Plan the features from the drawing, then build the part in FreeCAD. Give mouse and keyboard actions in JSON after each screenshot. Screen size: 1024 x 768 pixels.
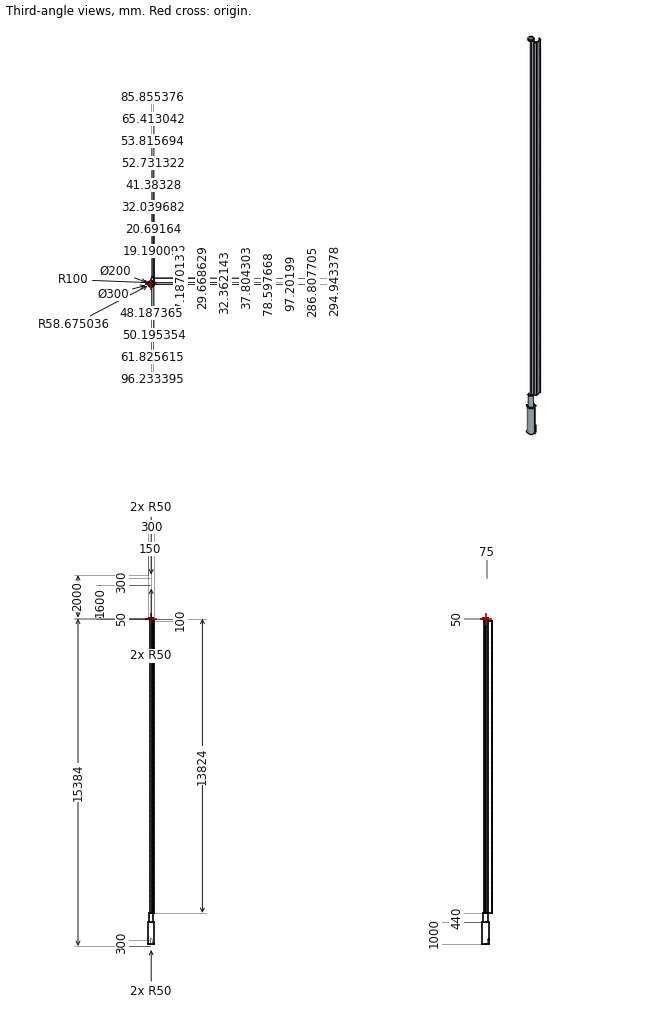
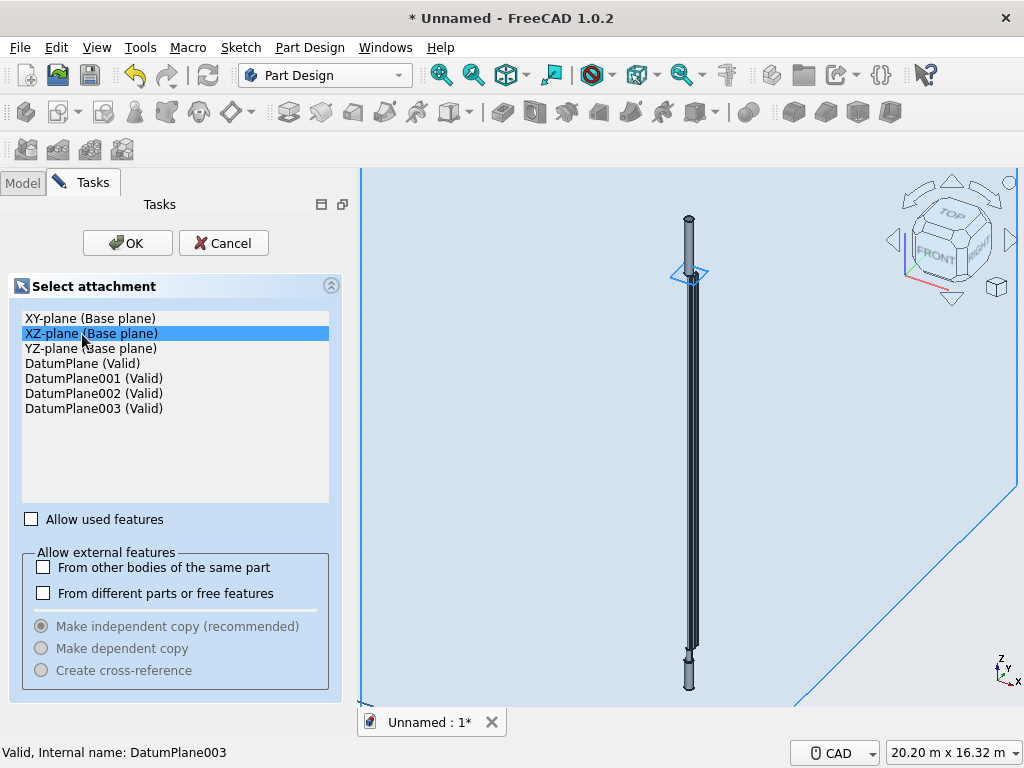
{"action": "left_click", "coordinate": [128, 243]}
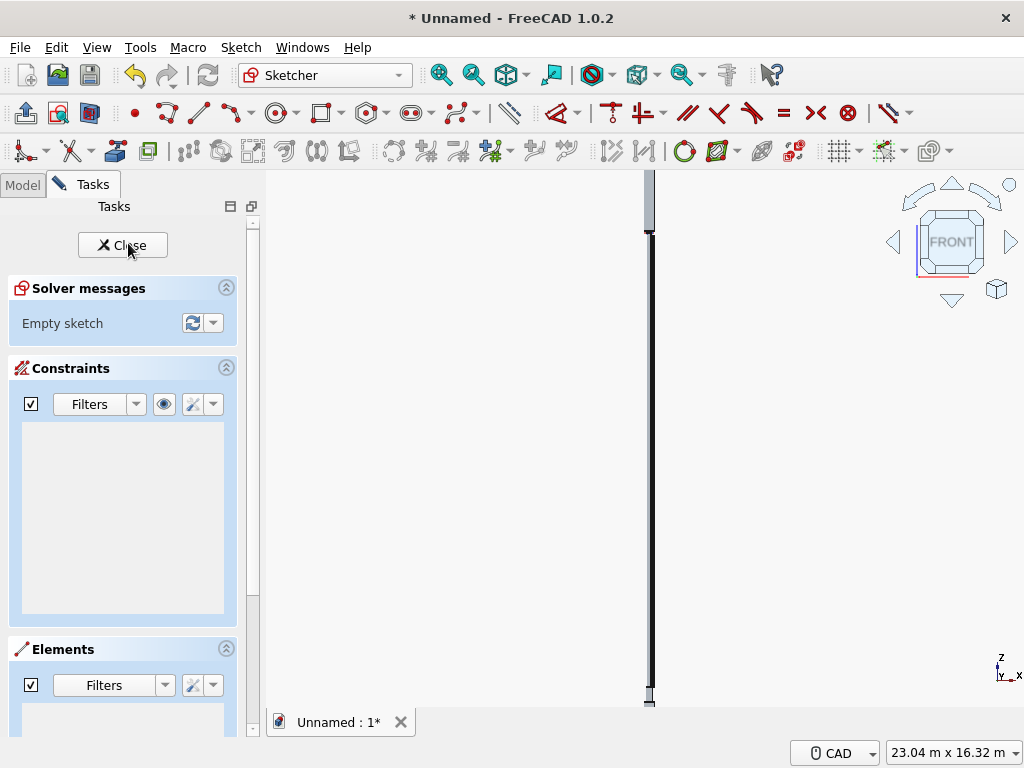
{"action": "left_click", "coordinate": [90, 114]}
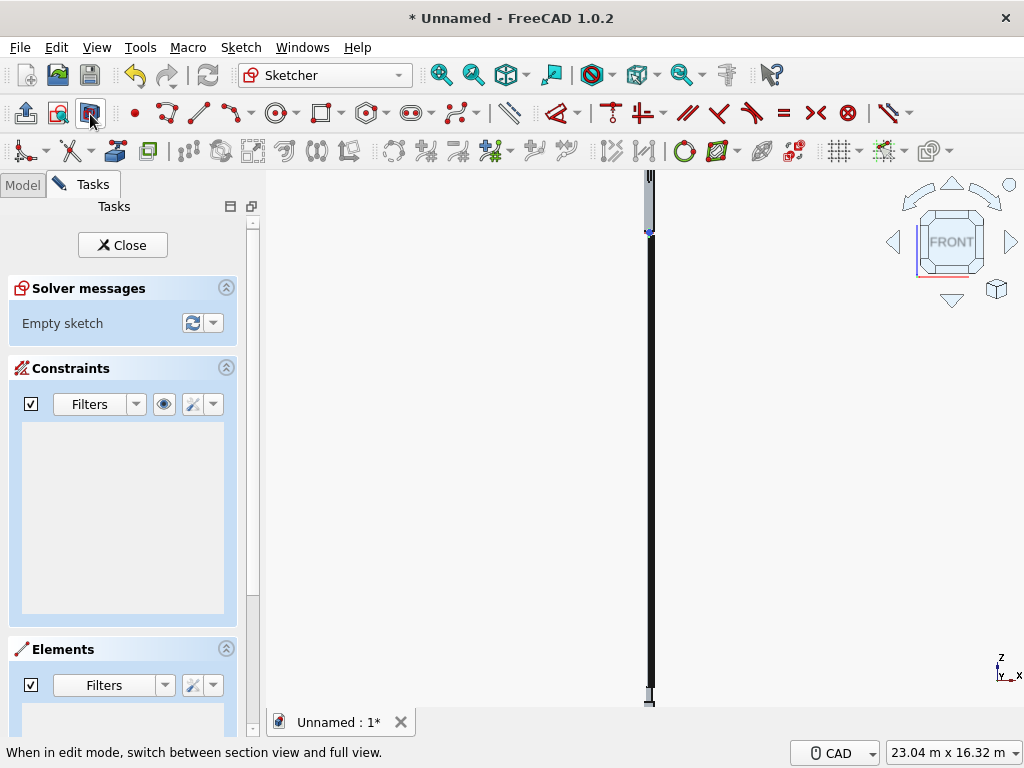
{"action": "scroll", "coordinate": [576, 438], "scroll_direction": "down", "scroll_amount": 5}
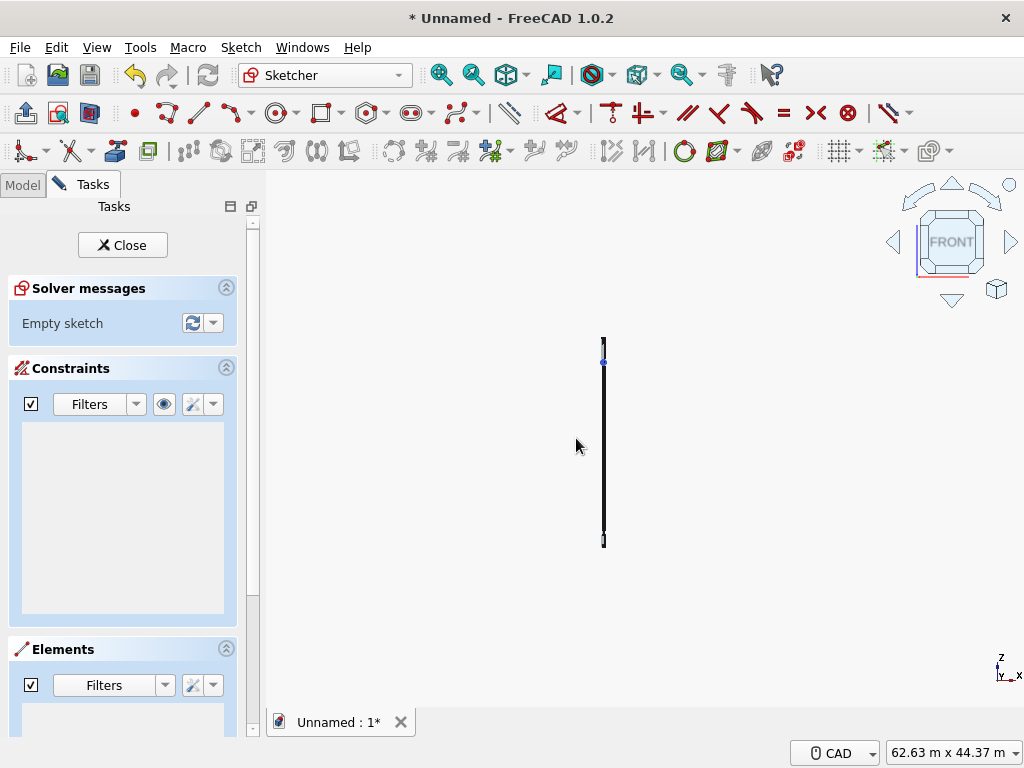
{"action": "scroll", "coordinate": [605, 343], "scroll_direction": "up", "scroll_amount": 13}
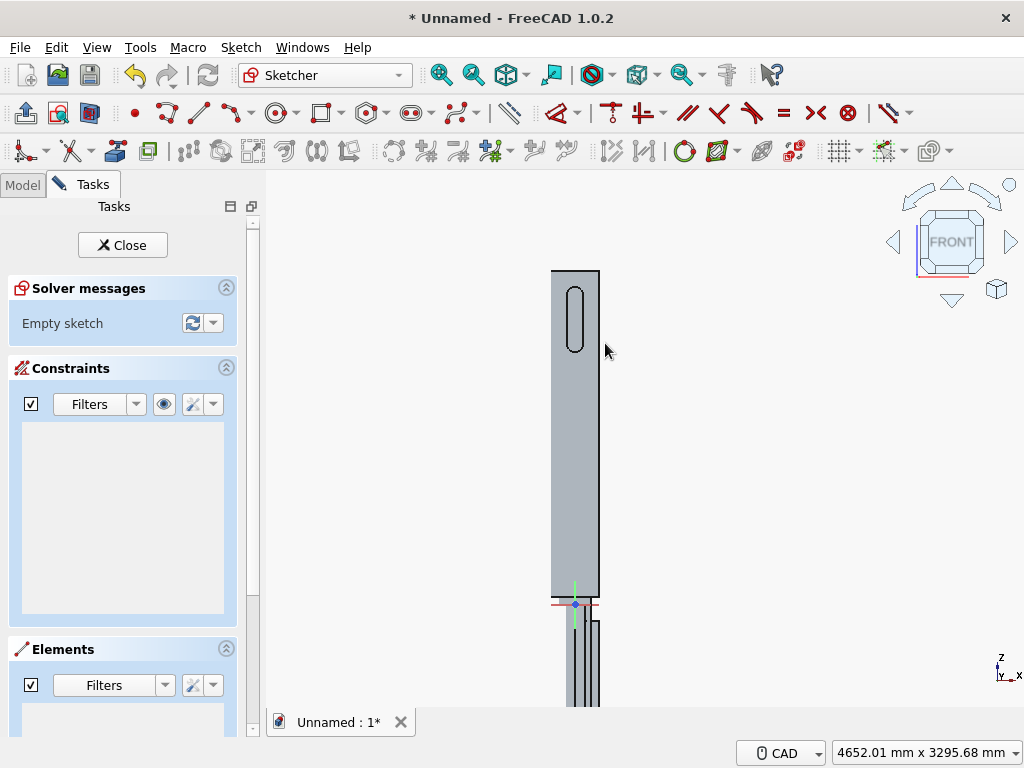
{"action": "left_click", "coordinate": [322, 114]}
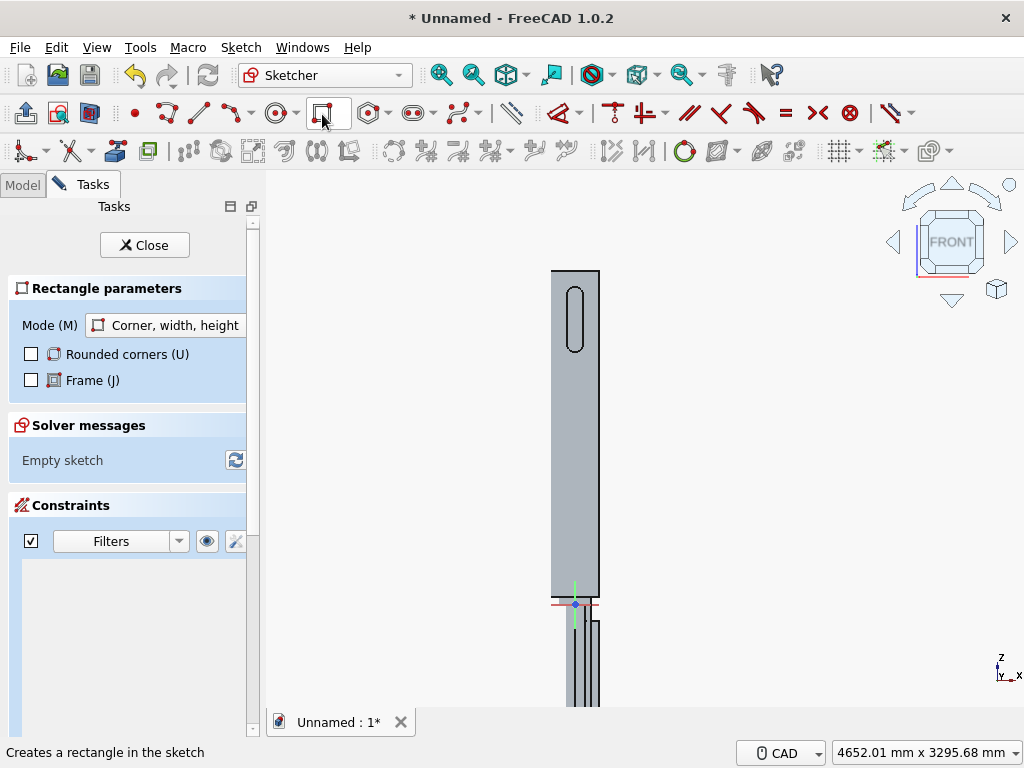
{"action": "left_click", "coordinate": [551, 271]}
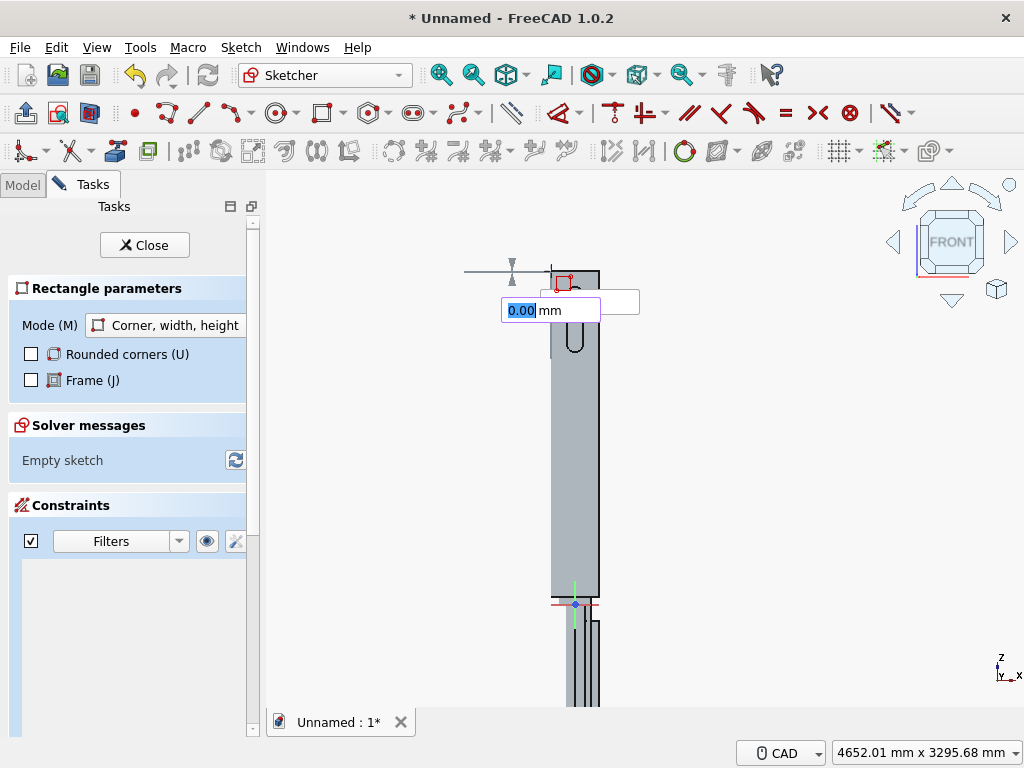
{"action": "scroll", "coordinate": [599, 597], "scroll_direction": "up", "scroll_amount": 4}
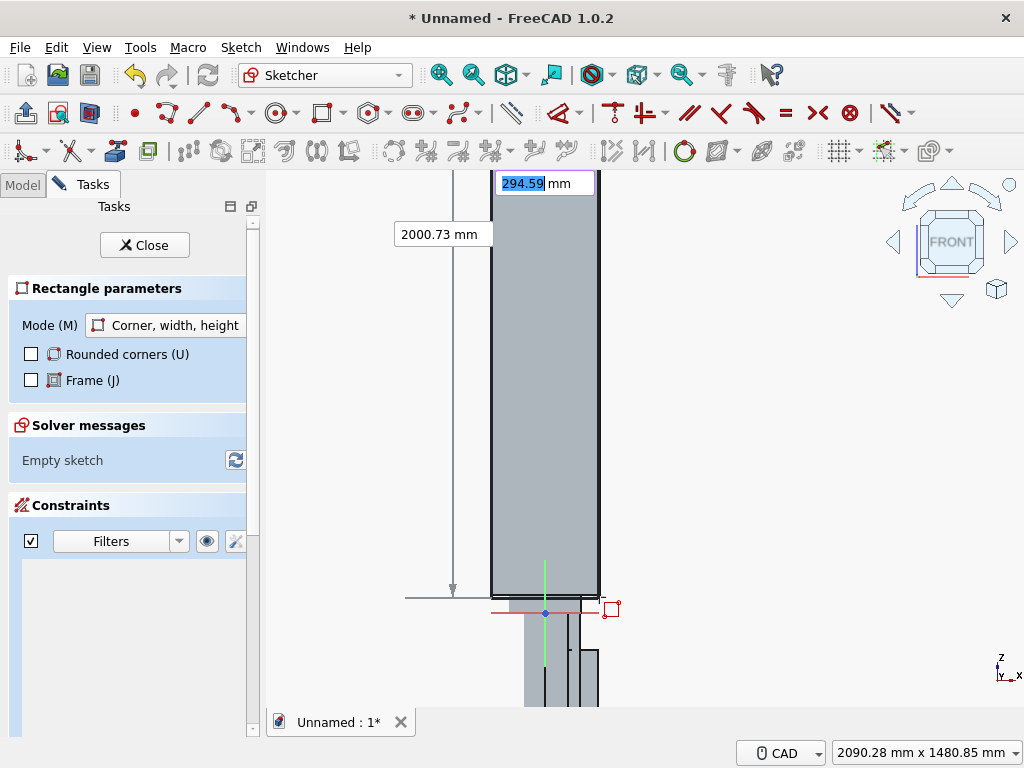
{"action": "left_click", "coordinate": [600, 595]}
{"action": "key", "text": "Escape"}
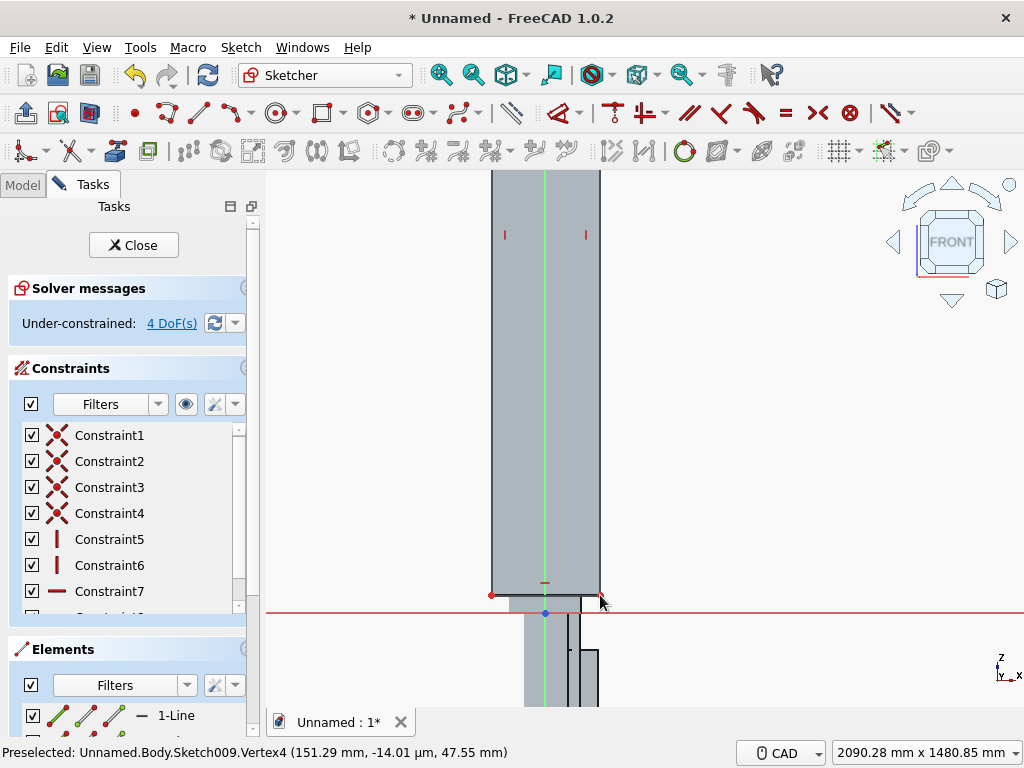
{"action": "left_click", "coordinate": [558, 114]}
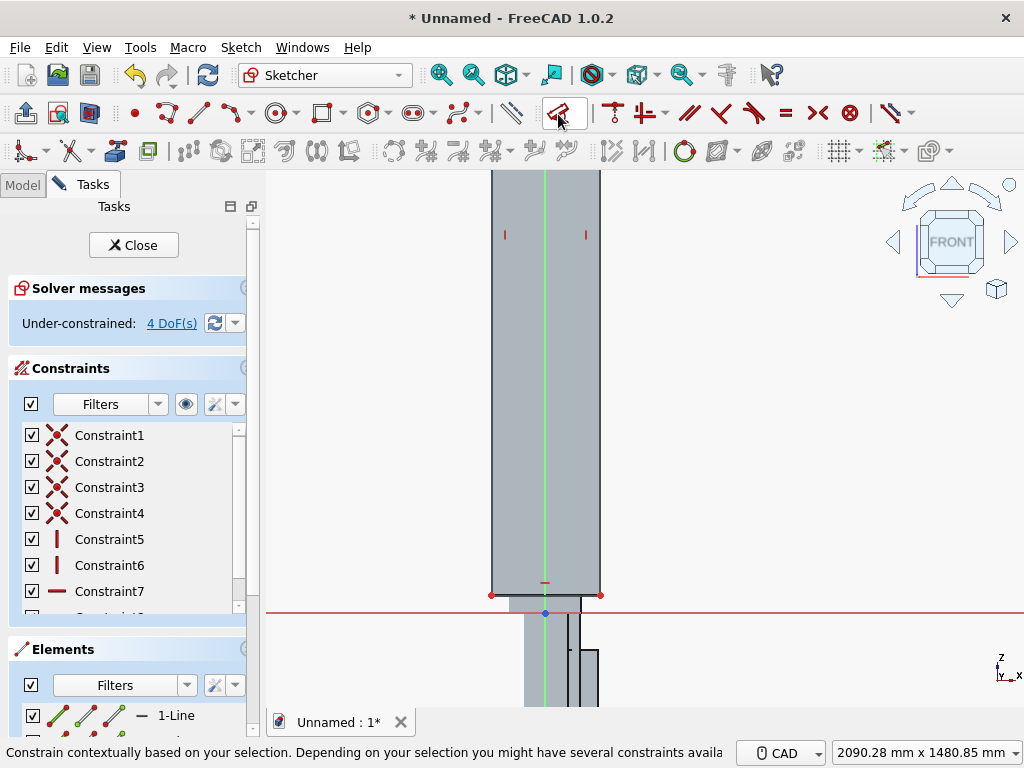
{"action": "left_click", "coordinate": [524, 596]}
{"action": "left_click", "coordinate": [521, 630]}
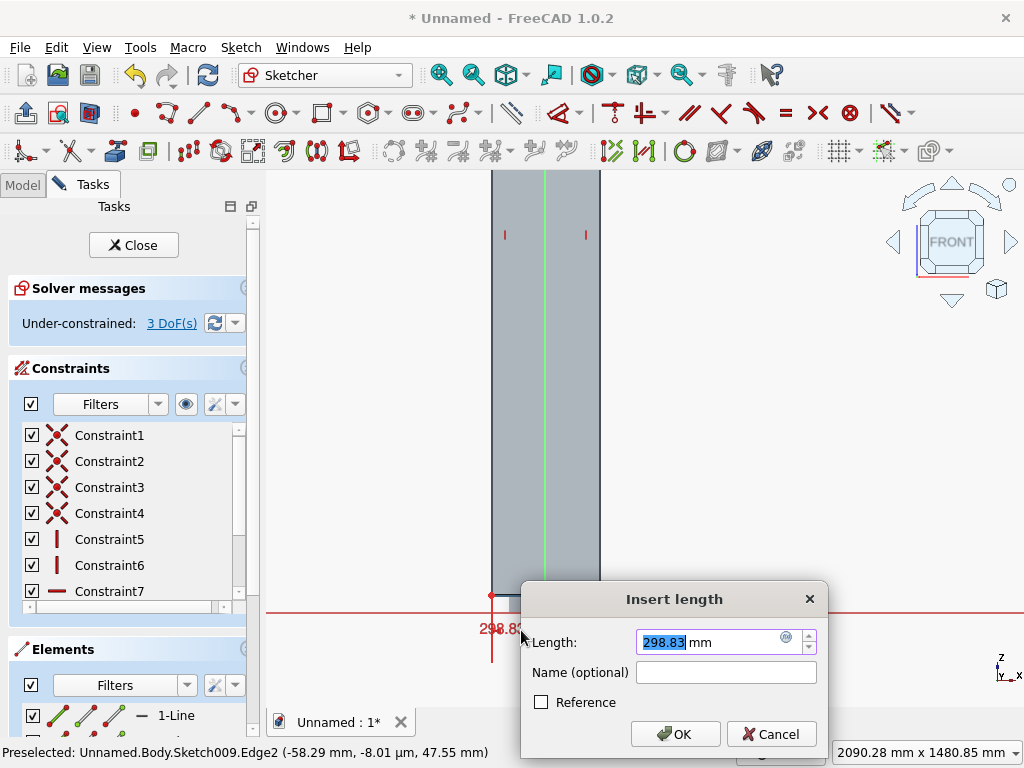
{"action": "type", "text": "300"}
{"action": "key", "text": "Return"}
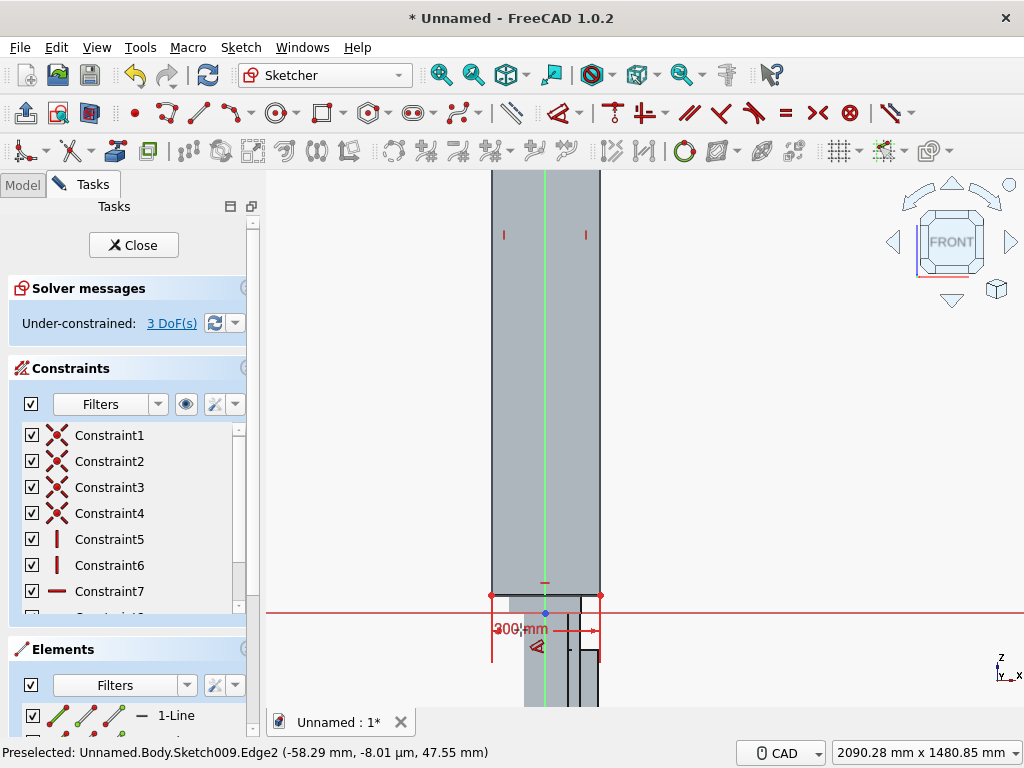
{"action": "scroll", "coordinate": [492, 596], "scroll_direction": "up", "scroll_amount": 4}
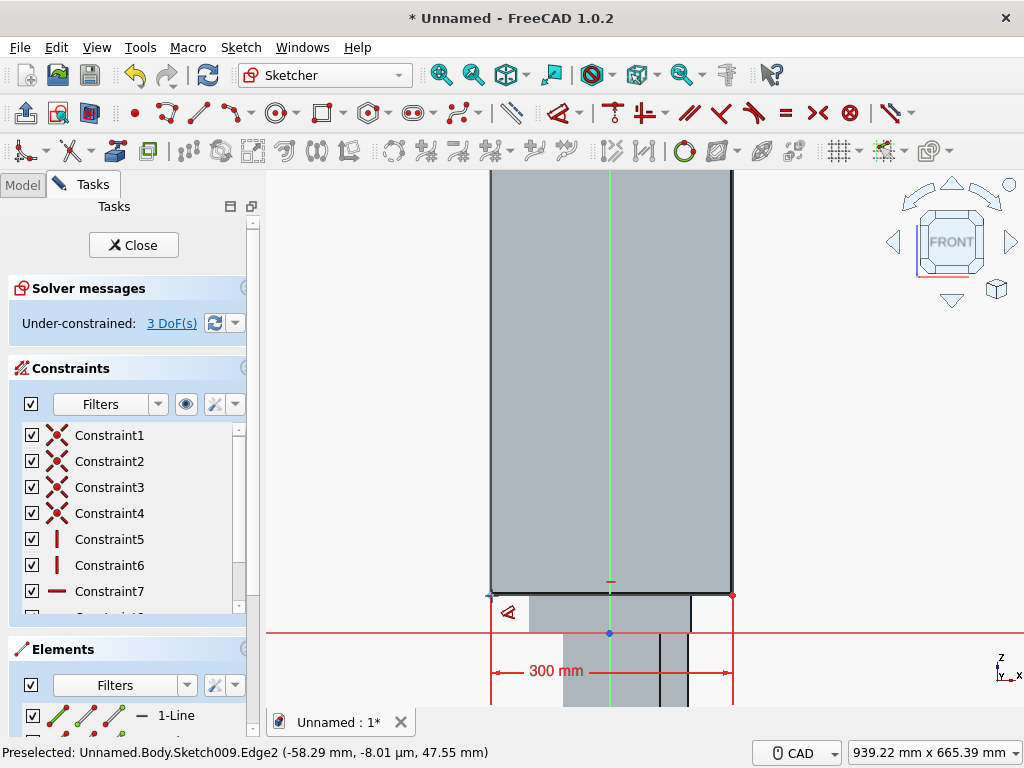
{"action": "left_click", "coordinate": [491, 595]}
{"action": "left_click", "coordinate": [457, 614]}